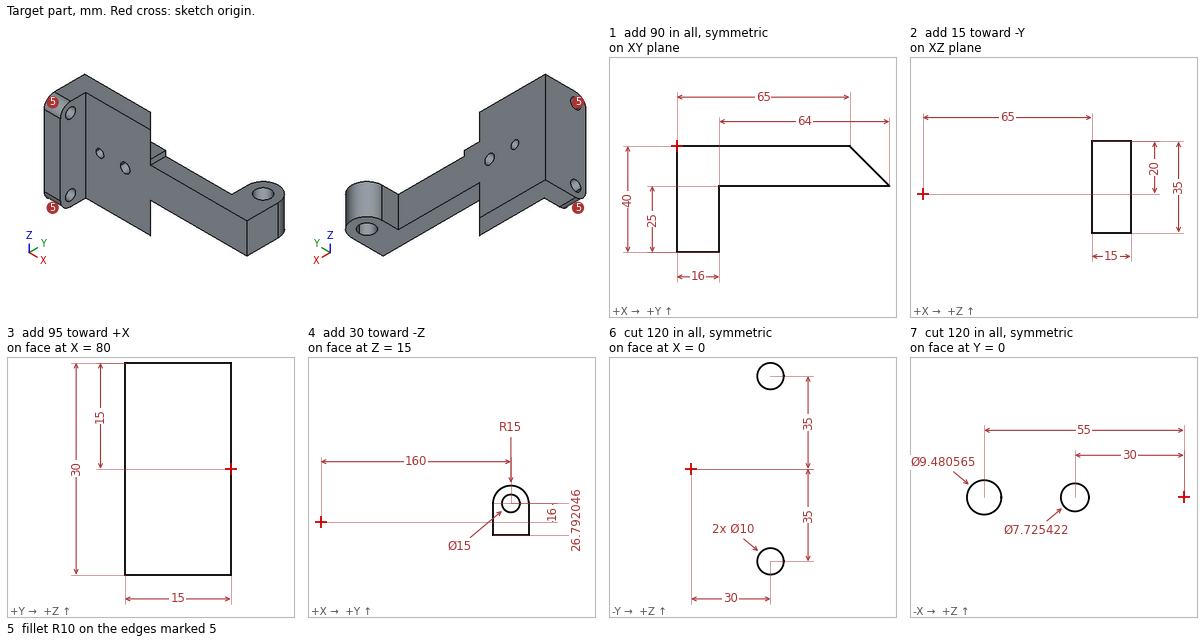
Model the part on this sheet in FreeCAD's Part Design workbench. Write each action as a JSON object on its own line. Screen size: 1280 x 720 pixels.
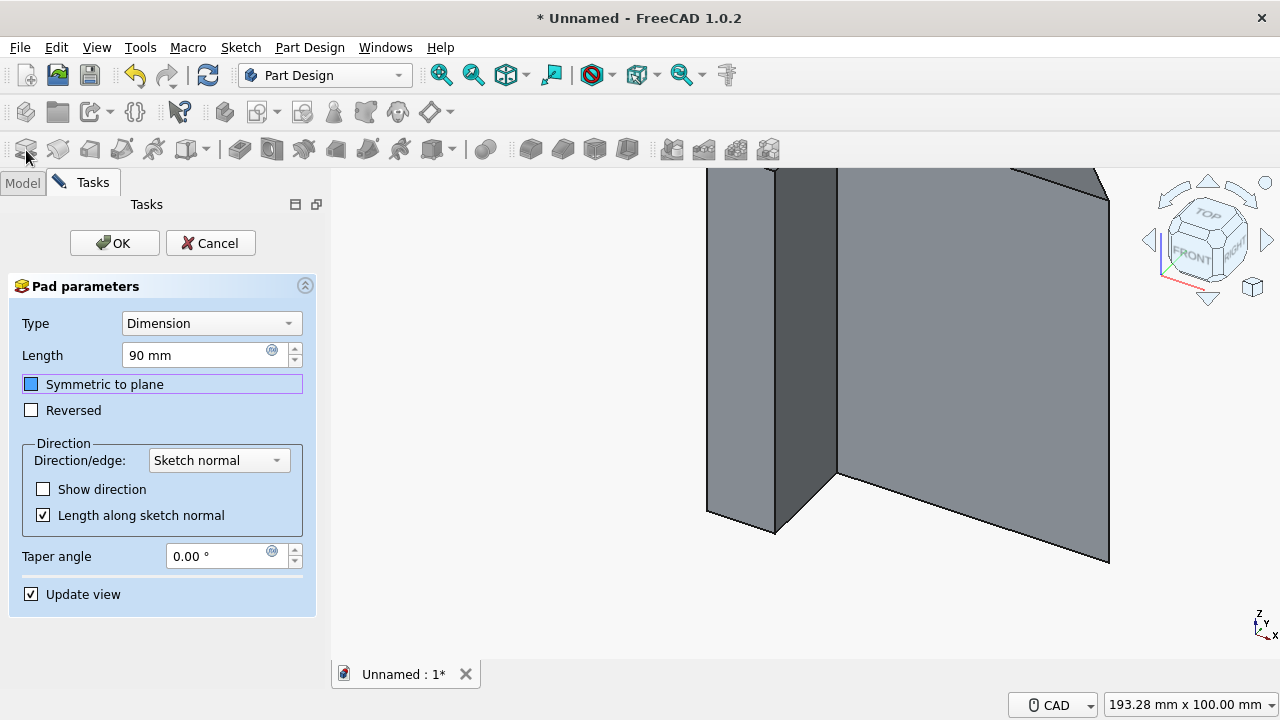
{"action": "left_click", "coordinate": [30, 384]}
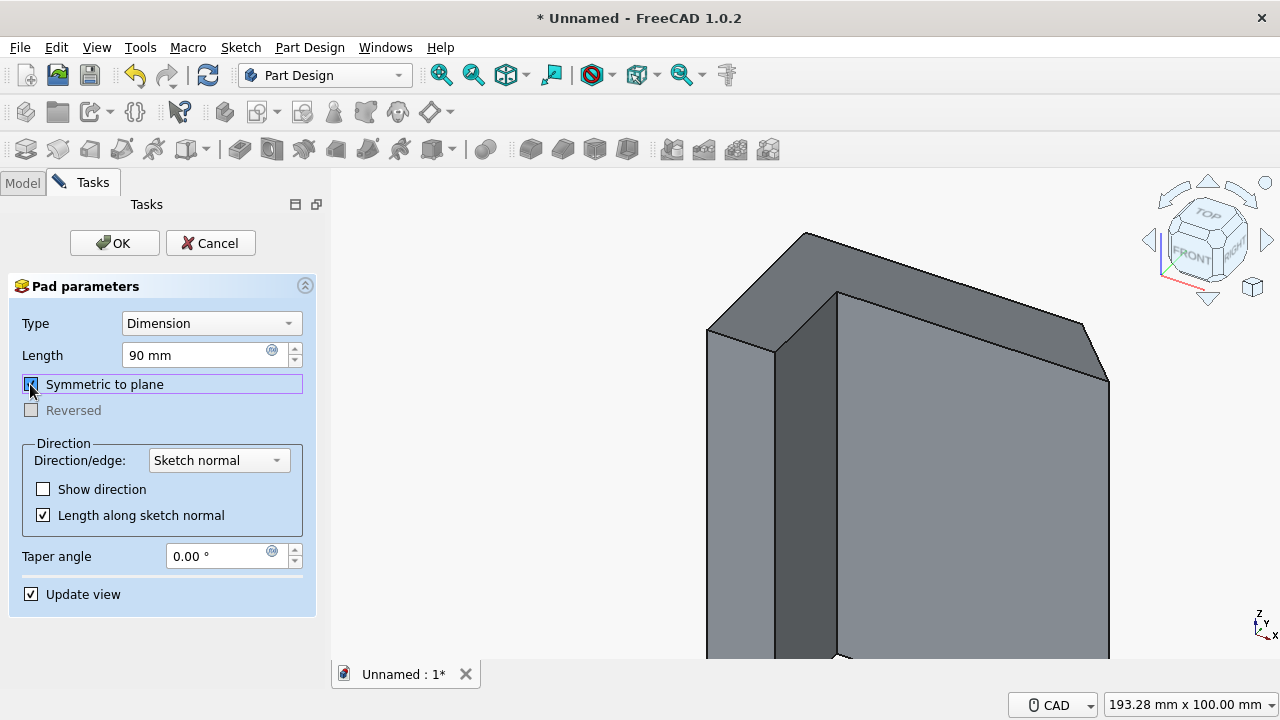
{"action": "left_click", "coordinate": [115, 243]}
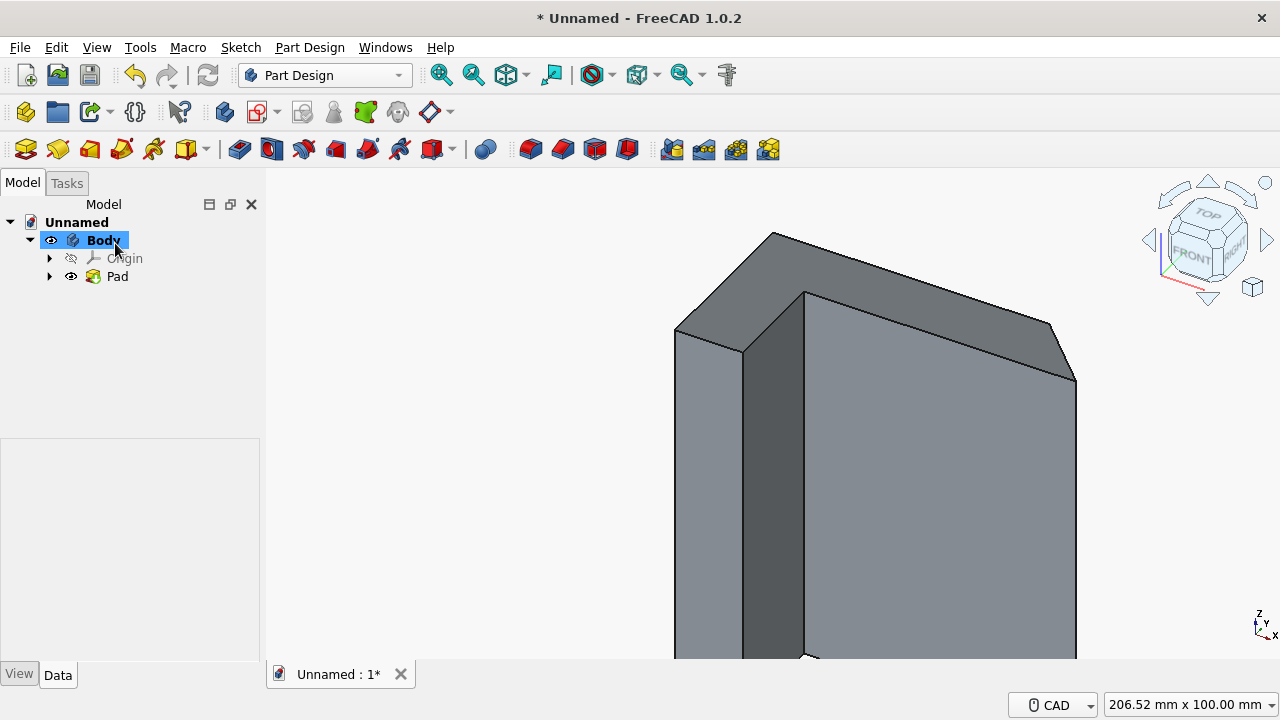
{"action": "left_click", "coordinate": [442, 76]}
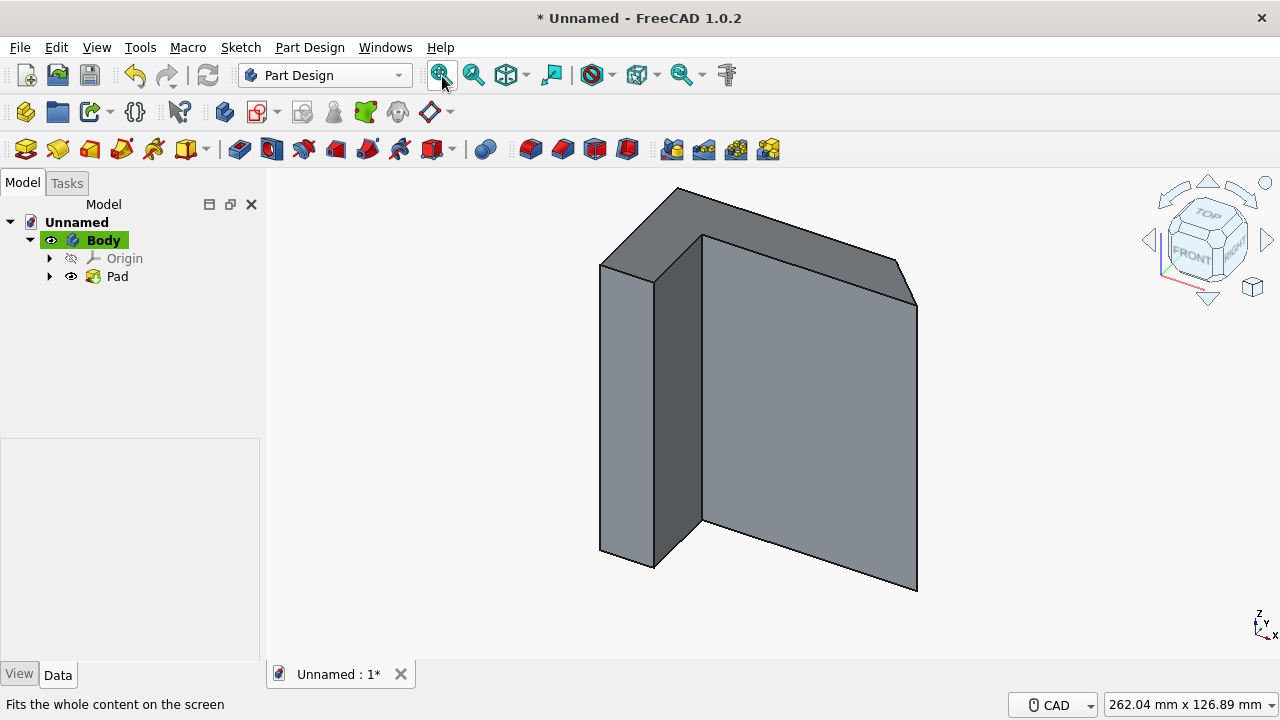
{"action": "left_click", "coordinate": [258, 112]}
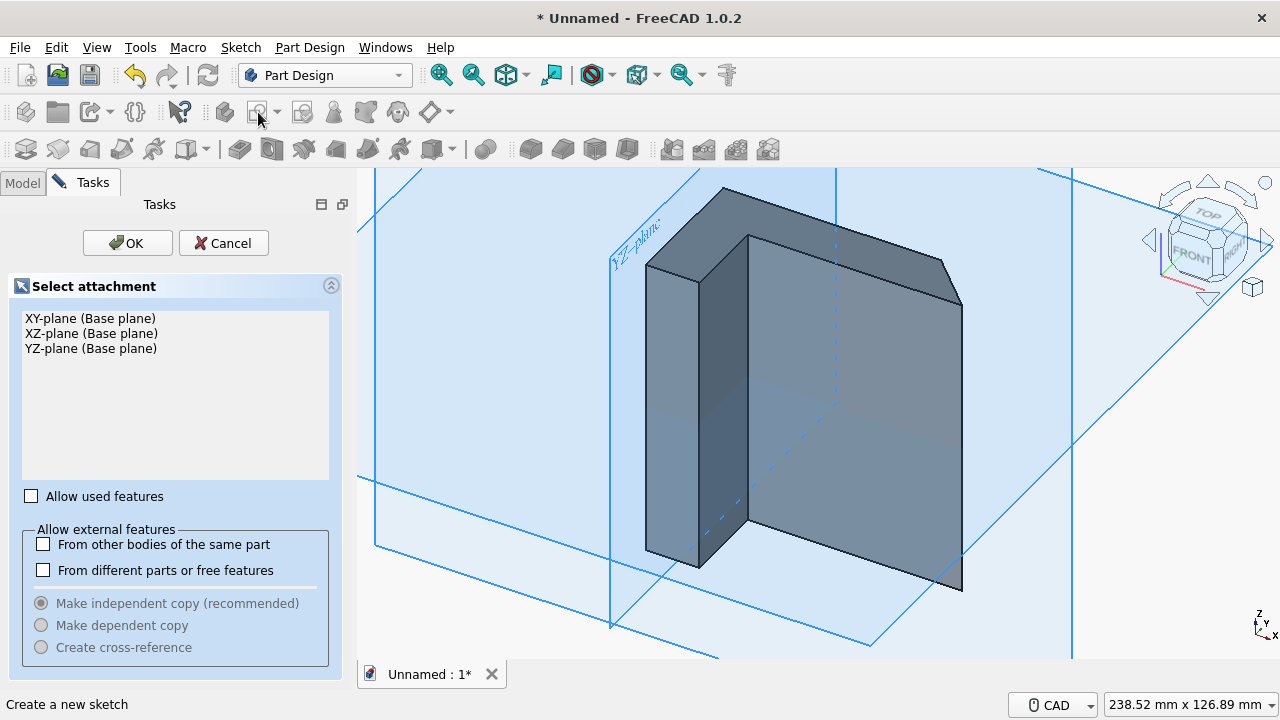
{"action": "left_click", "coordinate": [82, 334]}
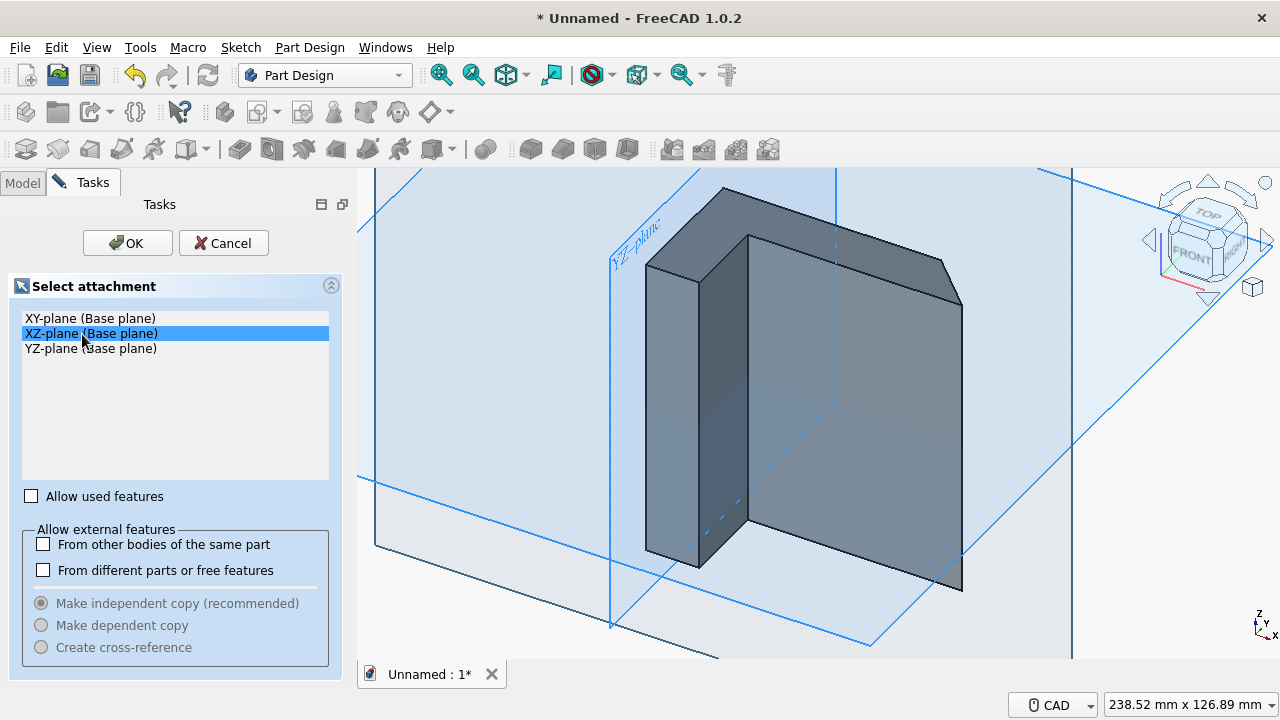
{"action": "left_click", "coordinate": [128, 243]}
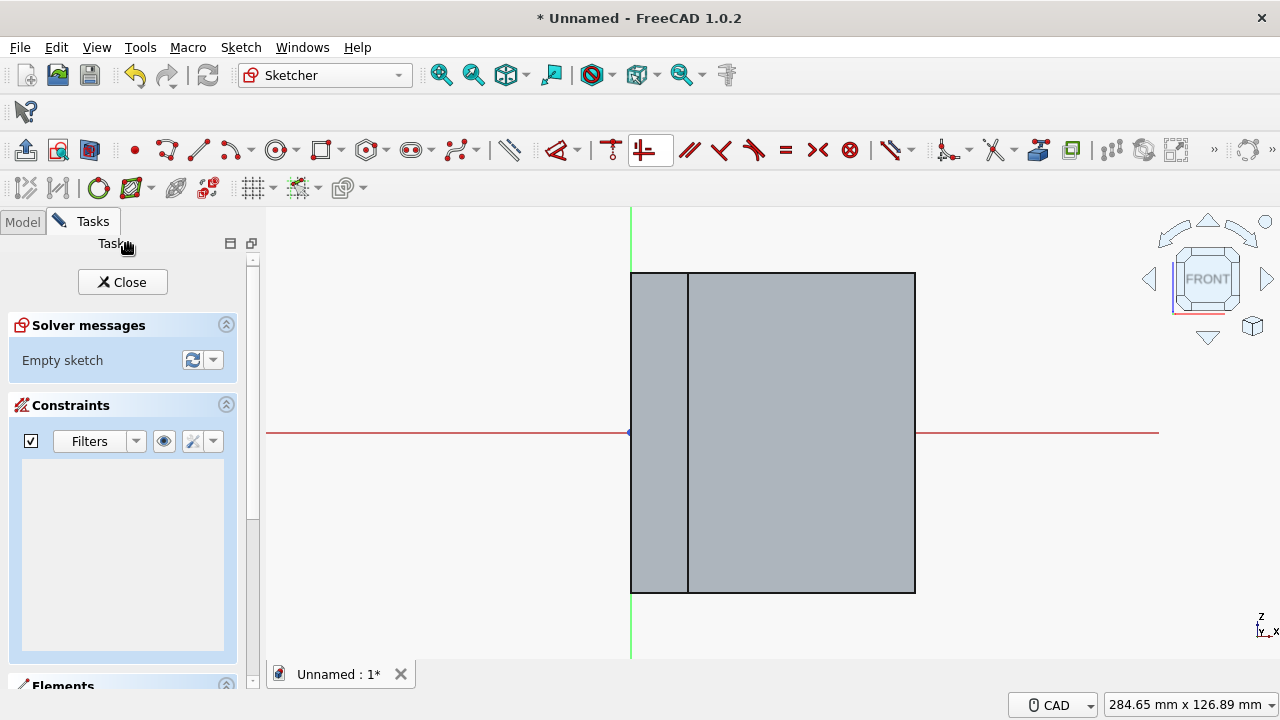
{"action": "left_click", "coordinate": [90, 150]}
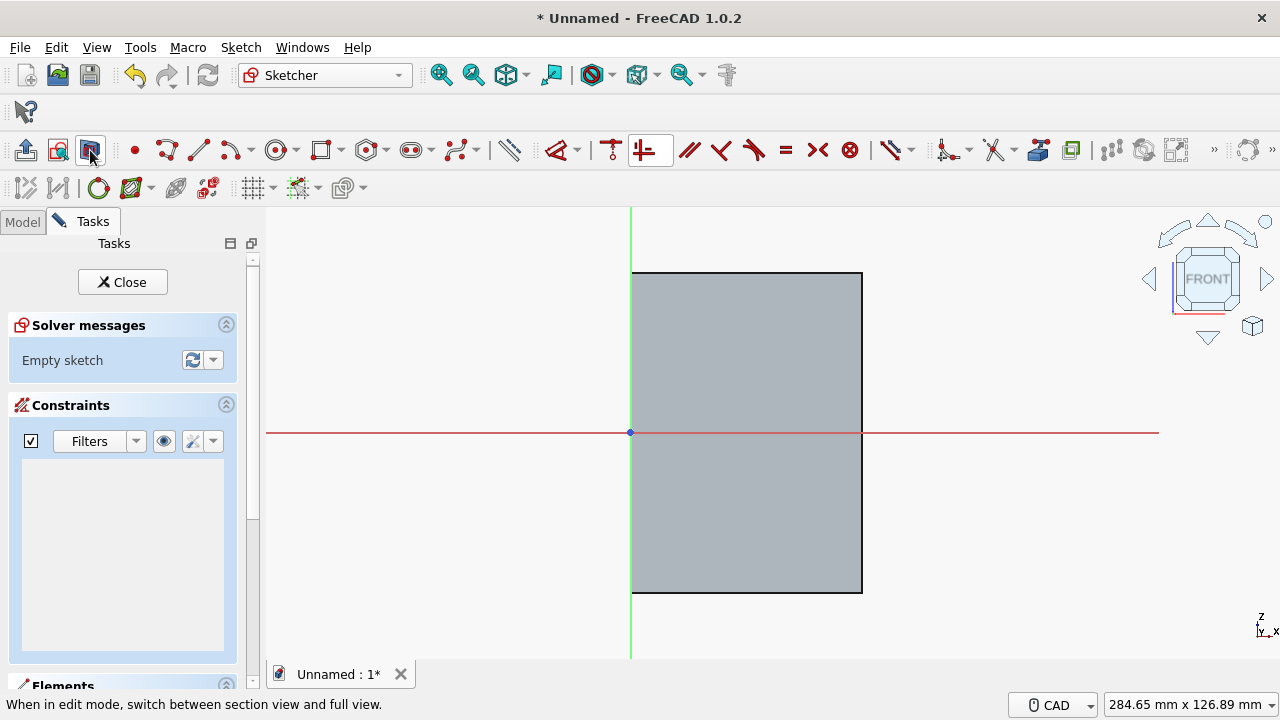
{"action": "scroll", "coordinate": [829, 417], "scroll_direction": "up", "scroll_amount": 4}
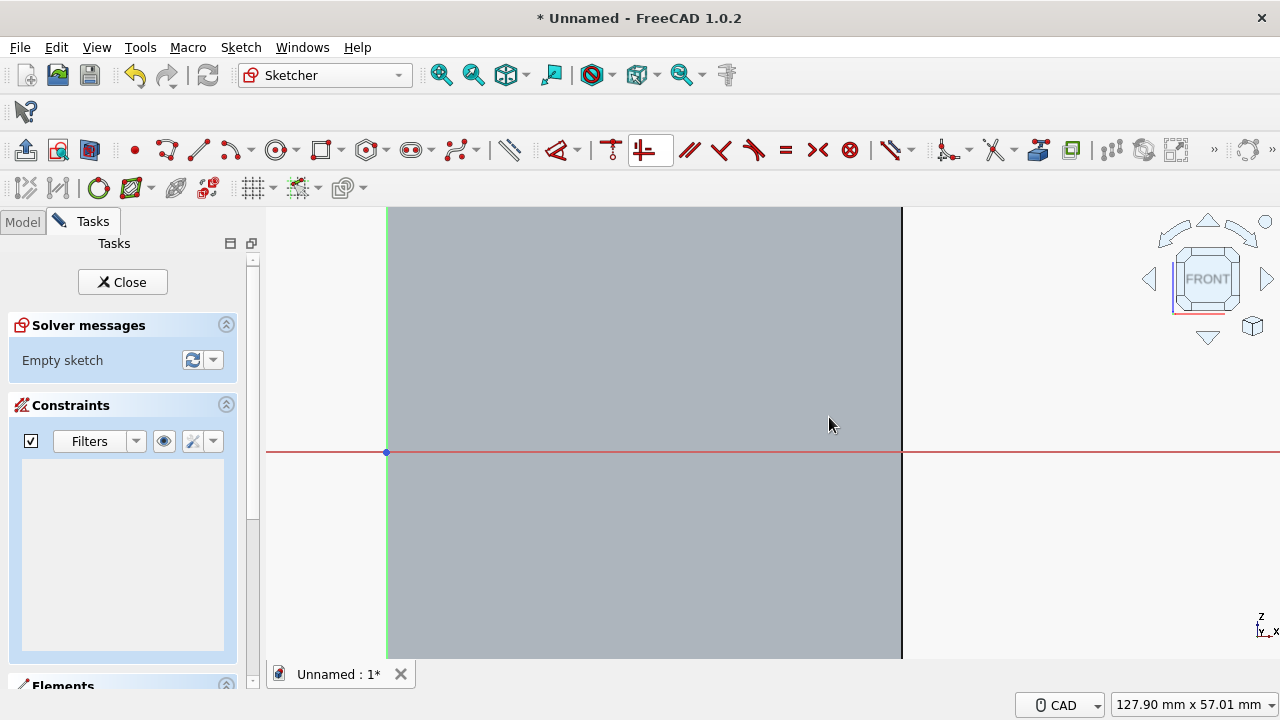
{"action": "left_click", "coordinate": [322, 150]}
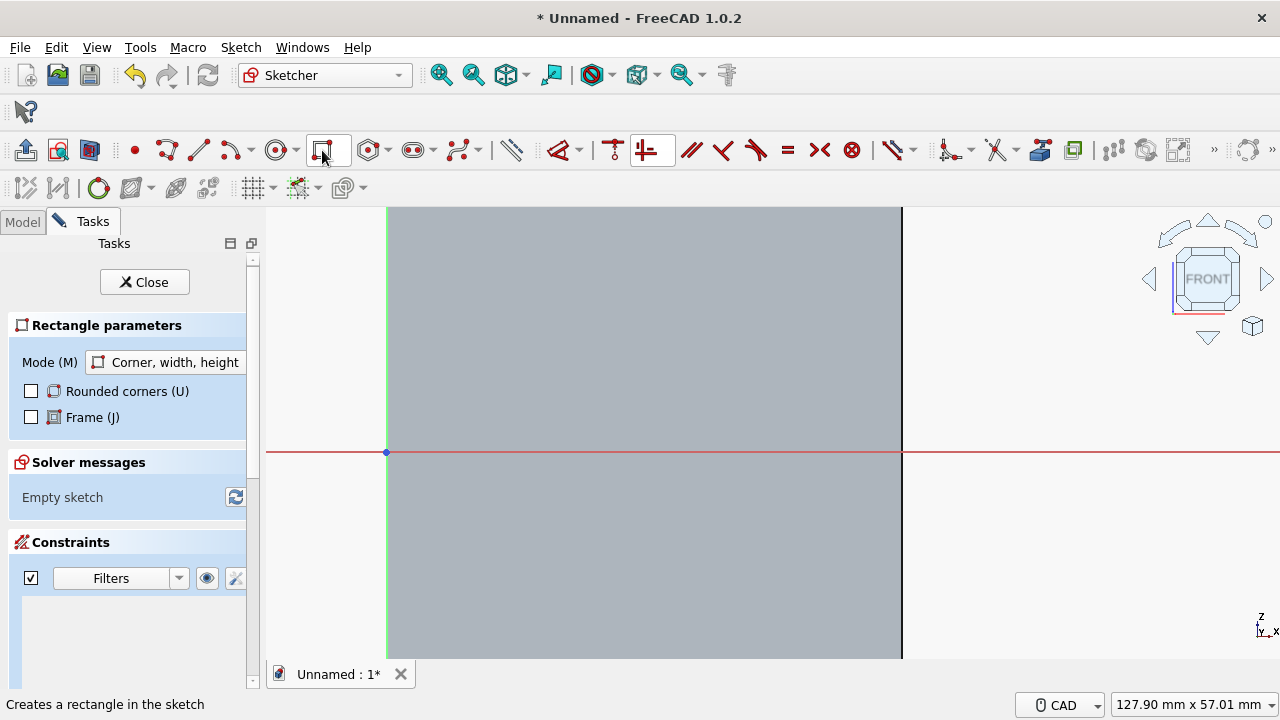
{"action": "left_click", "coordinate": [902, 293]}
{"action": "mouse_move", "coordinate": [1021, 571]}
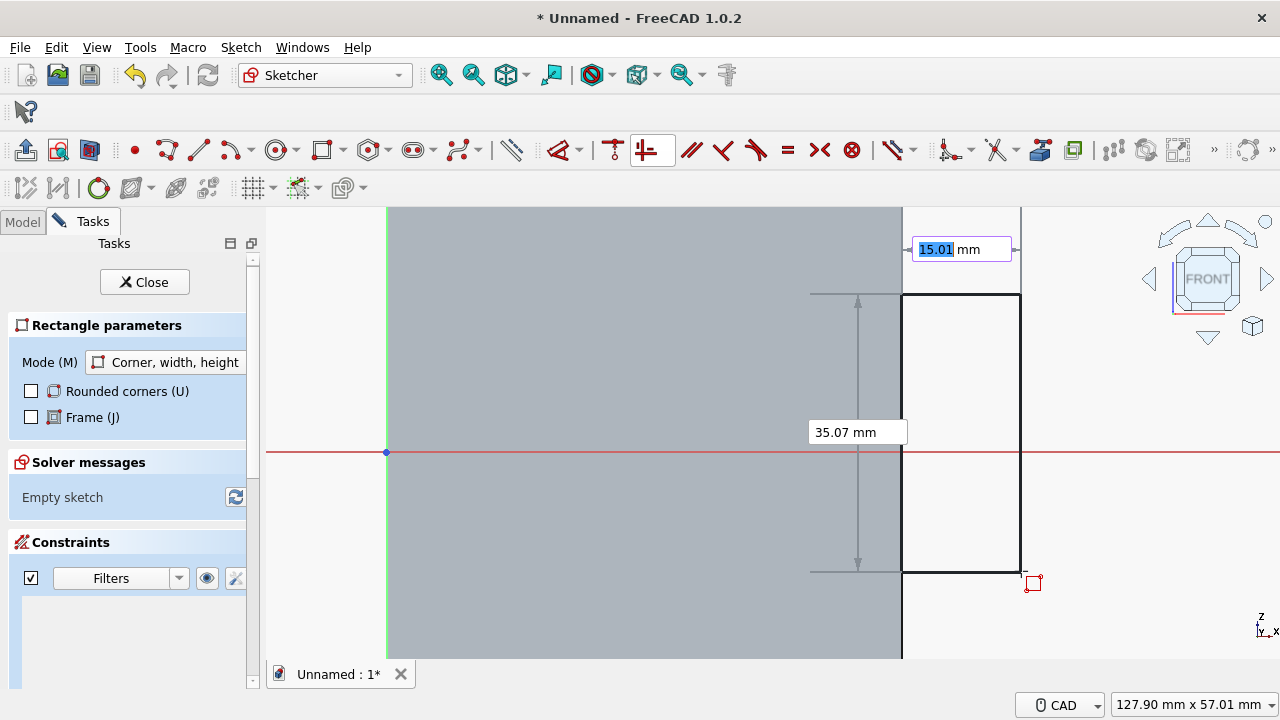
{"action": "type", "text": "15"}
{"action": "key", "text": "Tab"}
{"action": "type", "text": "35"}
{"action": "key", "text": "Return"}
{"action": "key", "text": "Escape"}